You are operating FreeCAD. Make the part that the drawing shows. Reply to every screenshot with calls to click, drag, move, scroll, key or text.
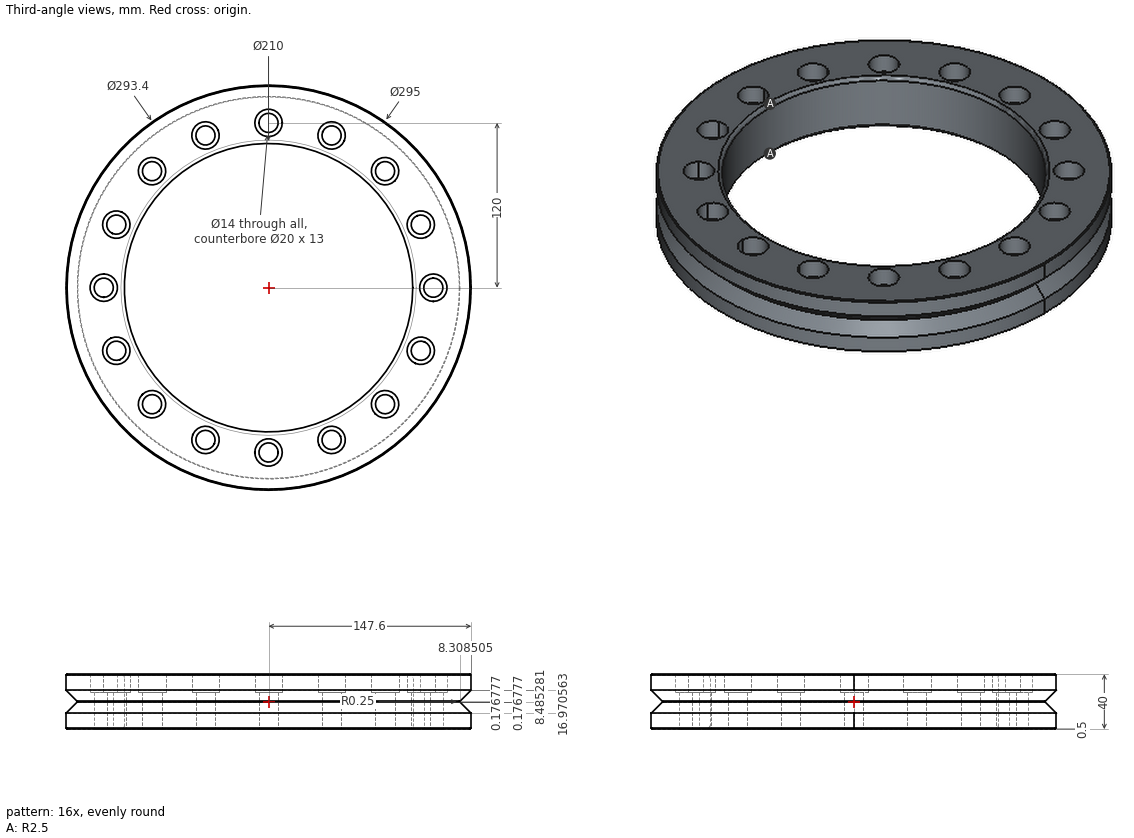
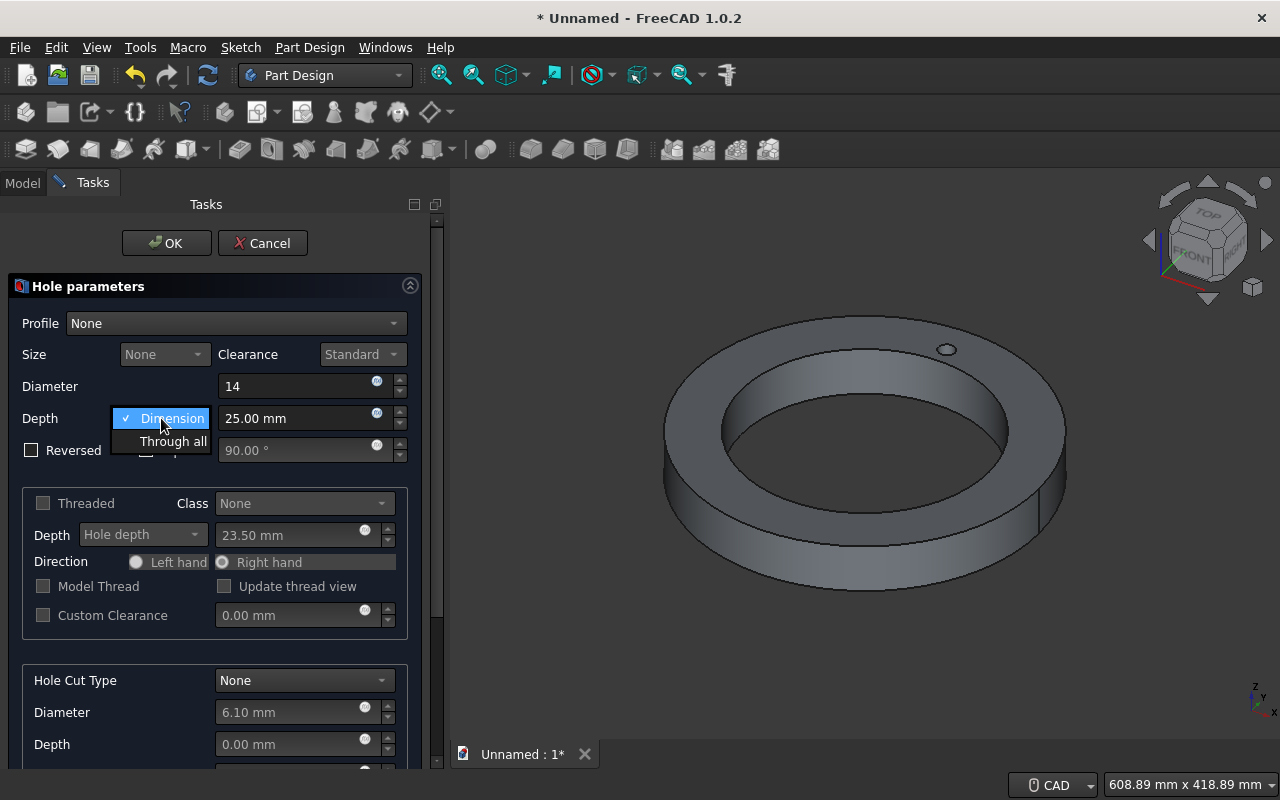
click(160, 442)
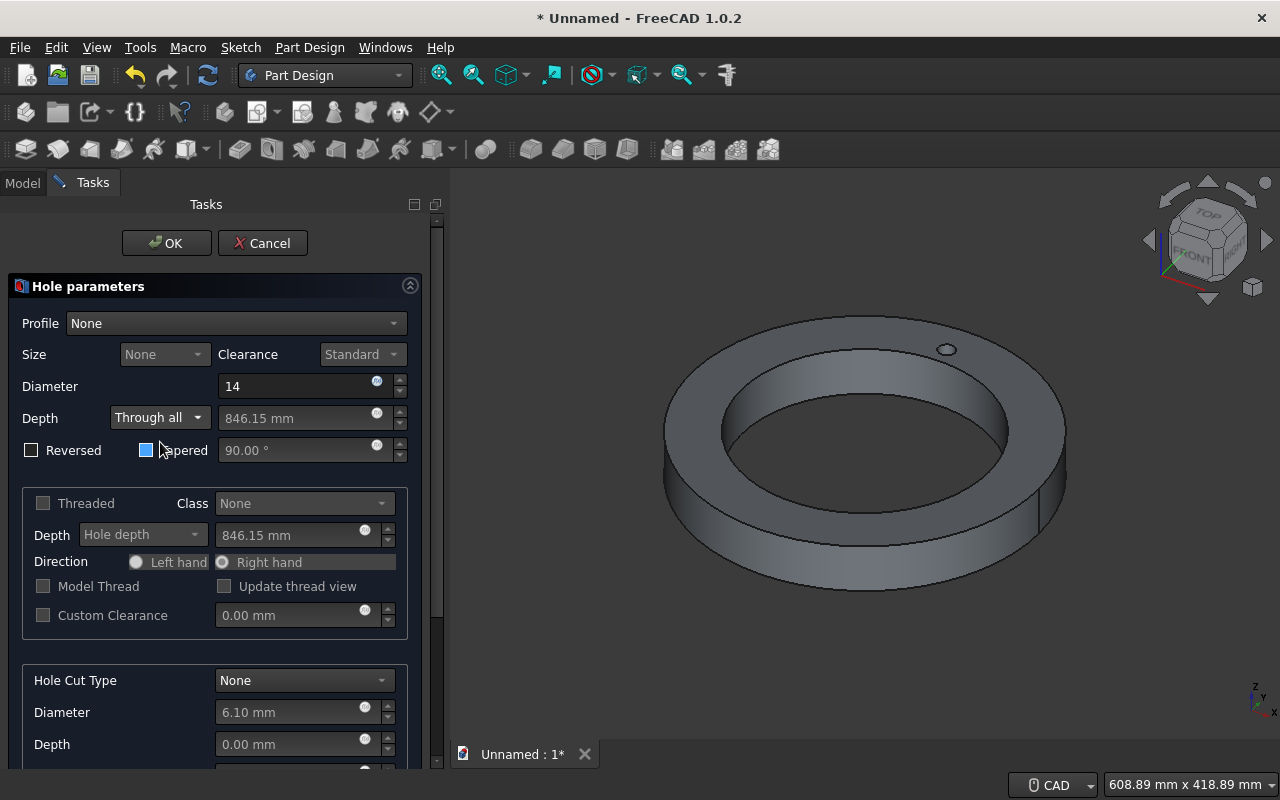
click(306, 680)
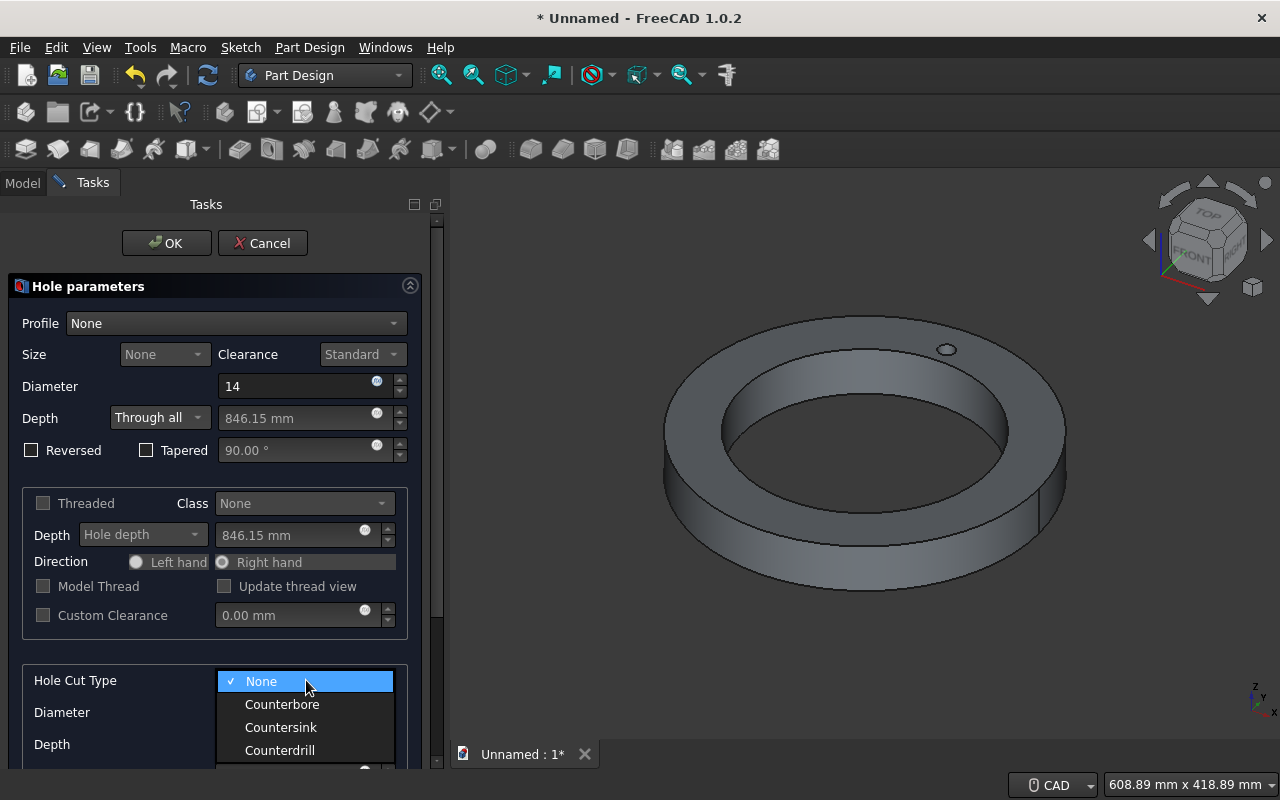
click(304, 704)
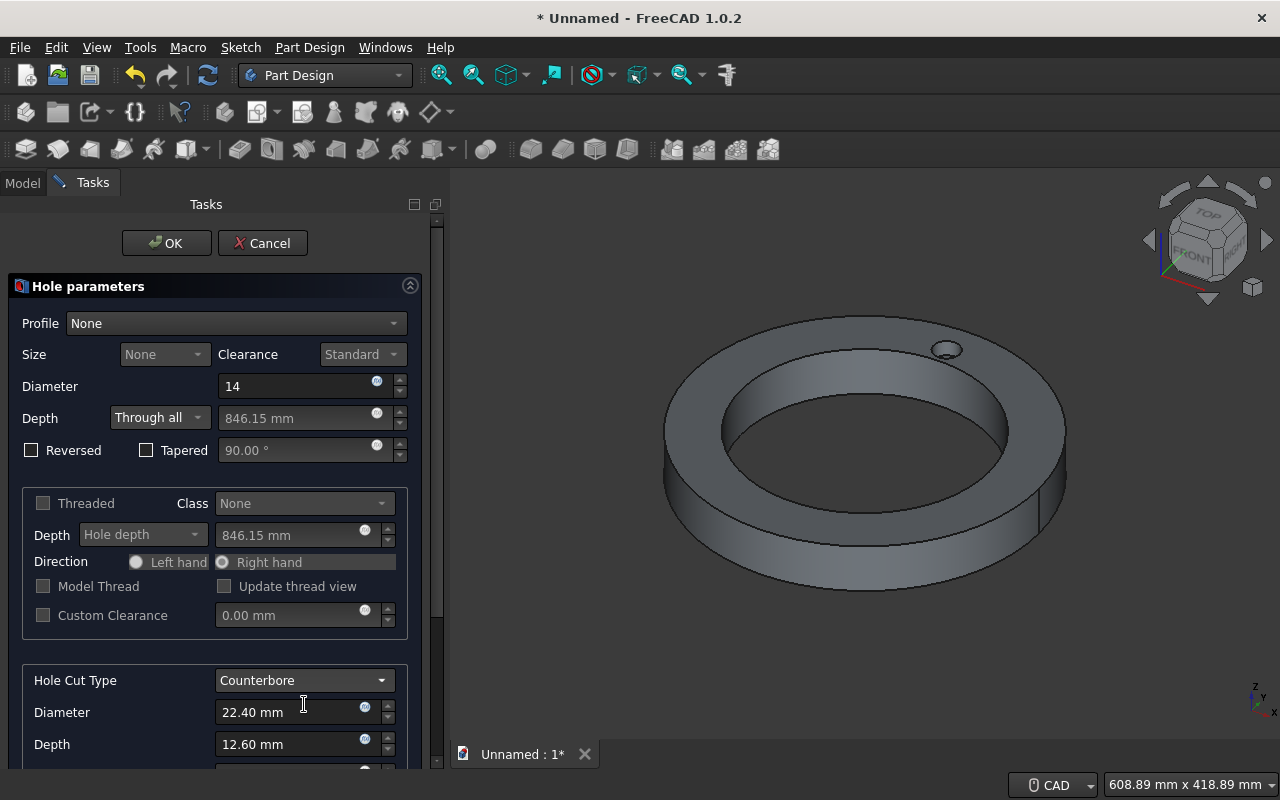
triple_click(298, 712)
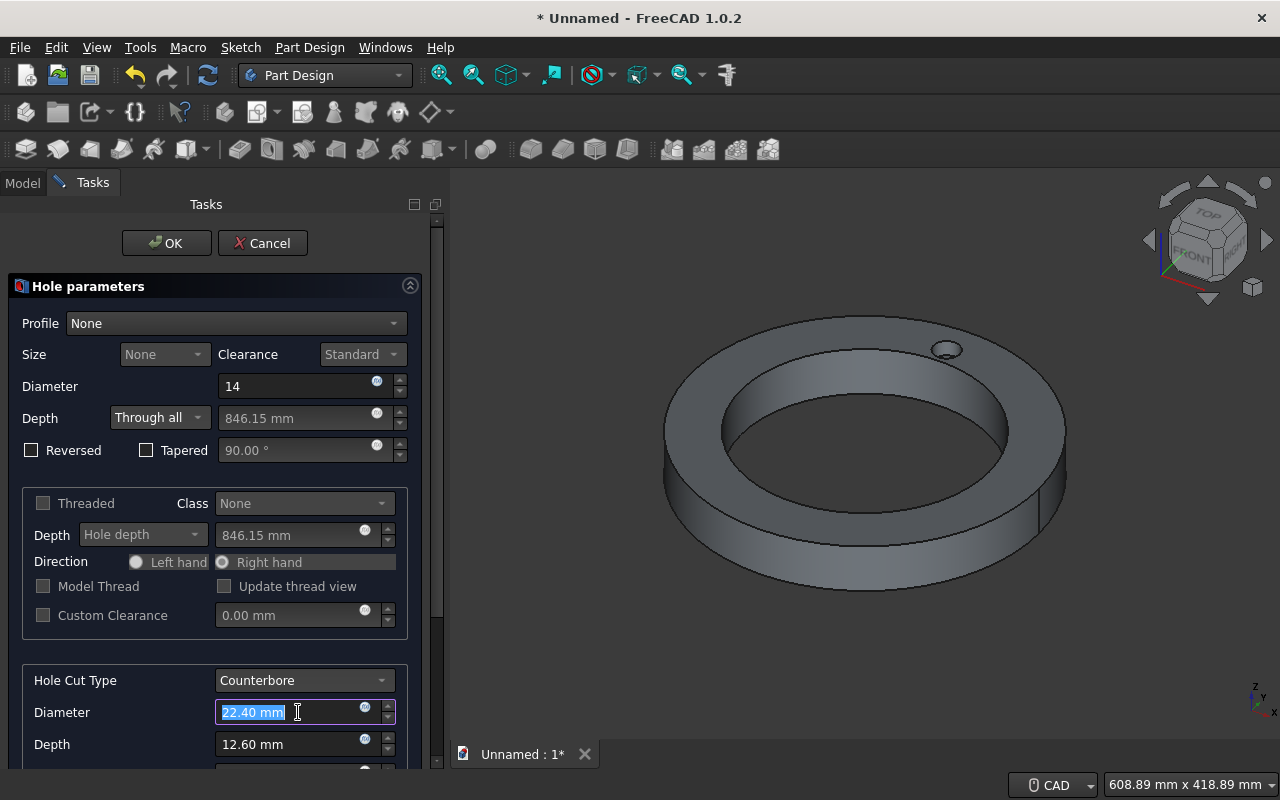
text(20)
key(Tab)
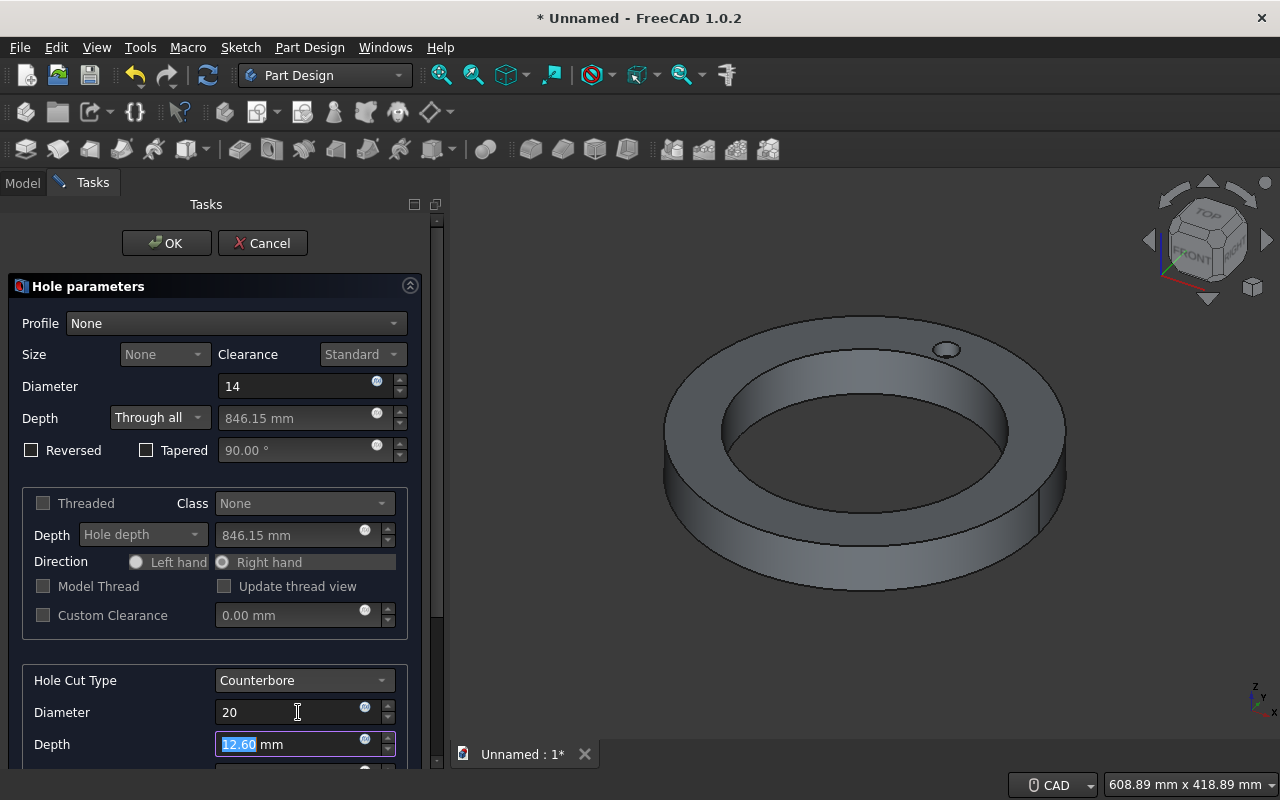
text(13)
key(Tab)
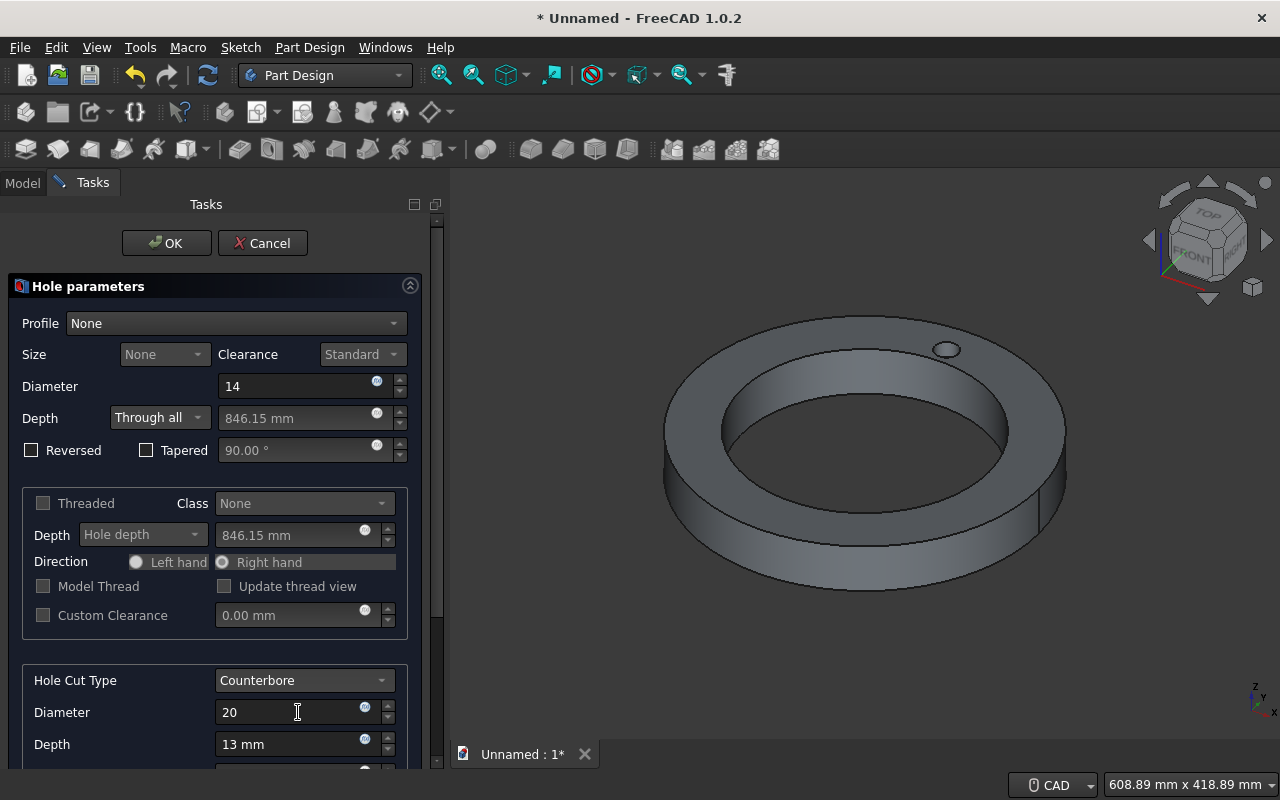
click(167, 243)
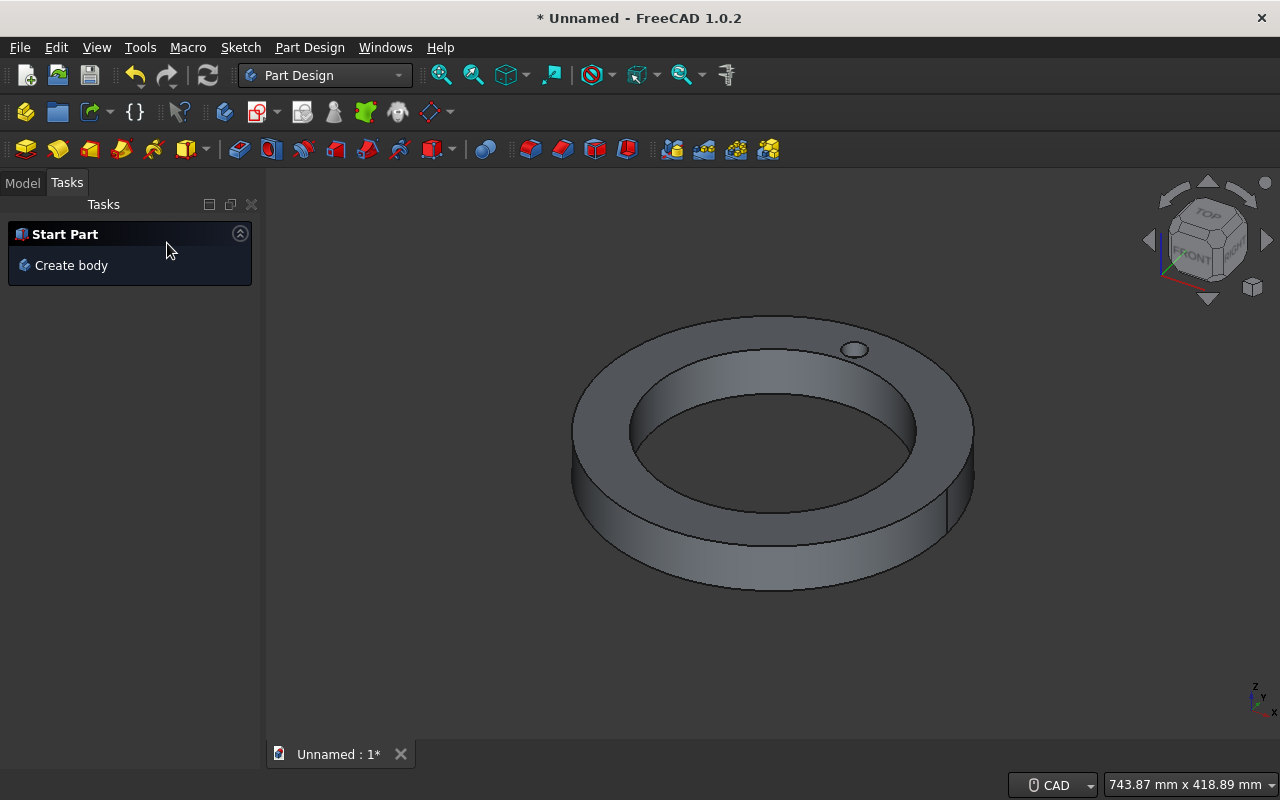
click(23, 182)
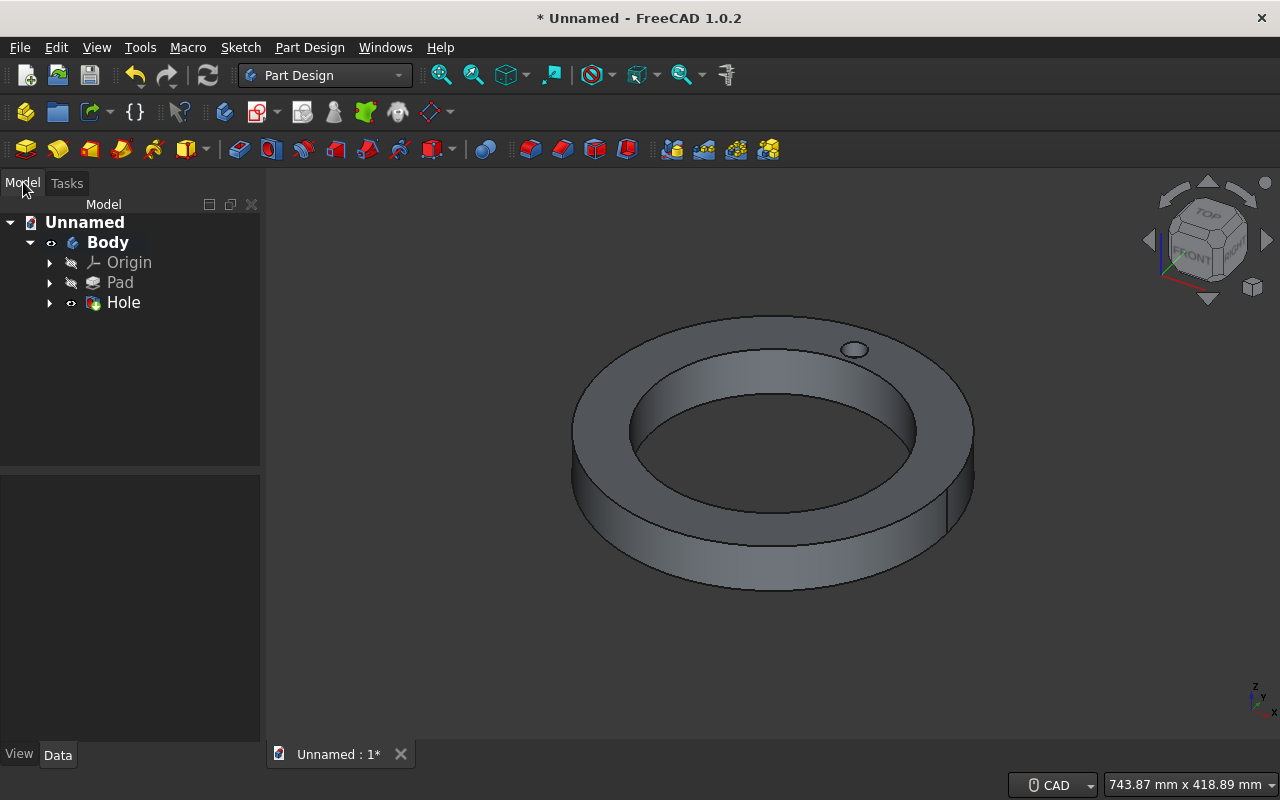
click(116, 303)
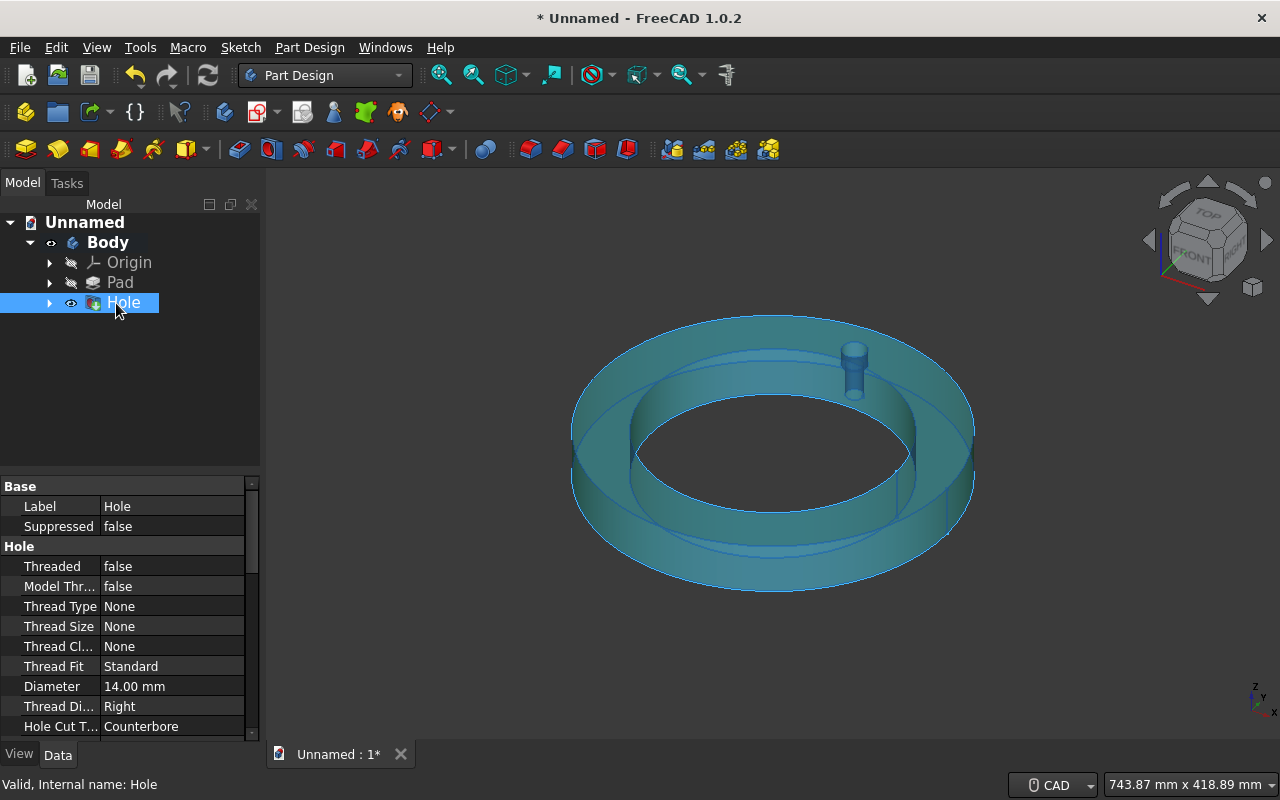
click(736, 150)